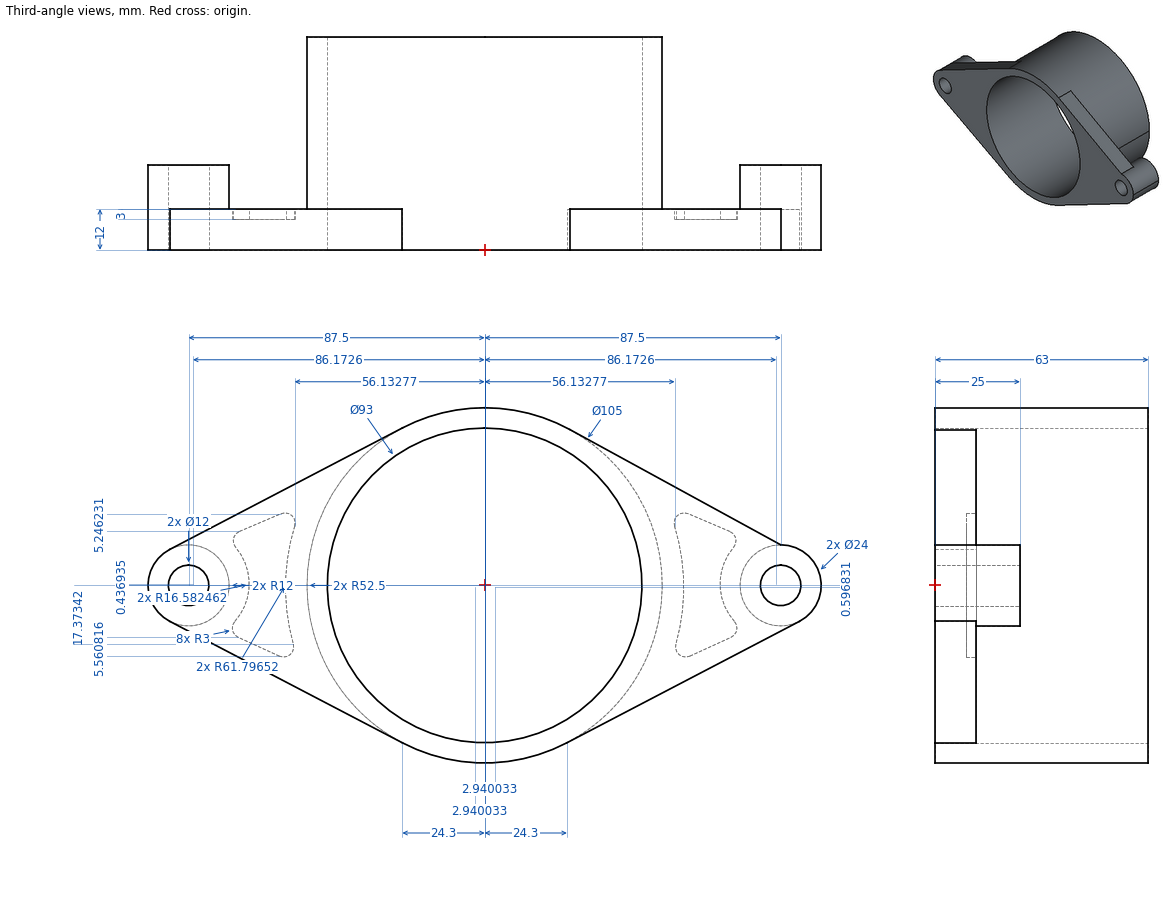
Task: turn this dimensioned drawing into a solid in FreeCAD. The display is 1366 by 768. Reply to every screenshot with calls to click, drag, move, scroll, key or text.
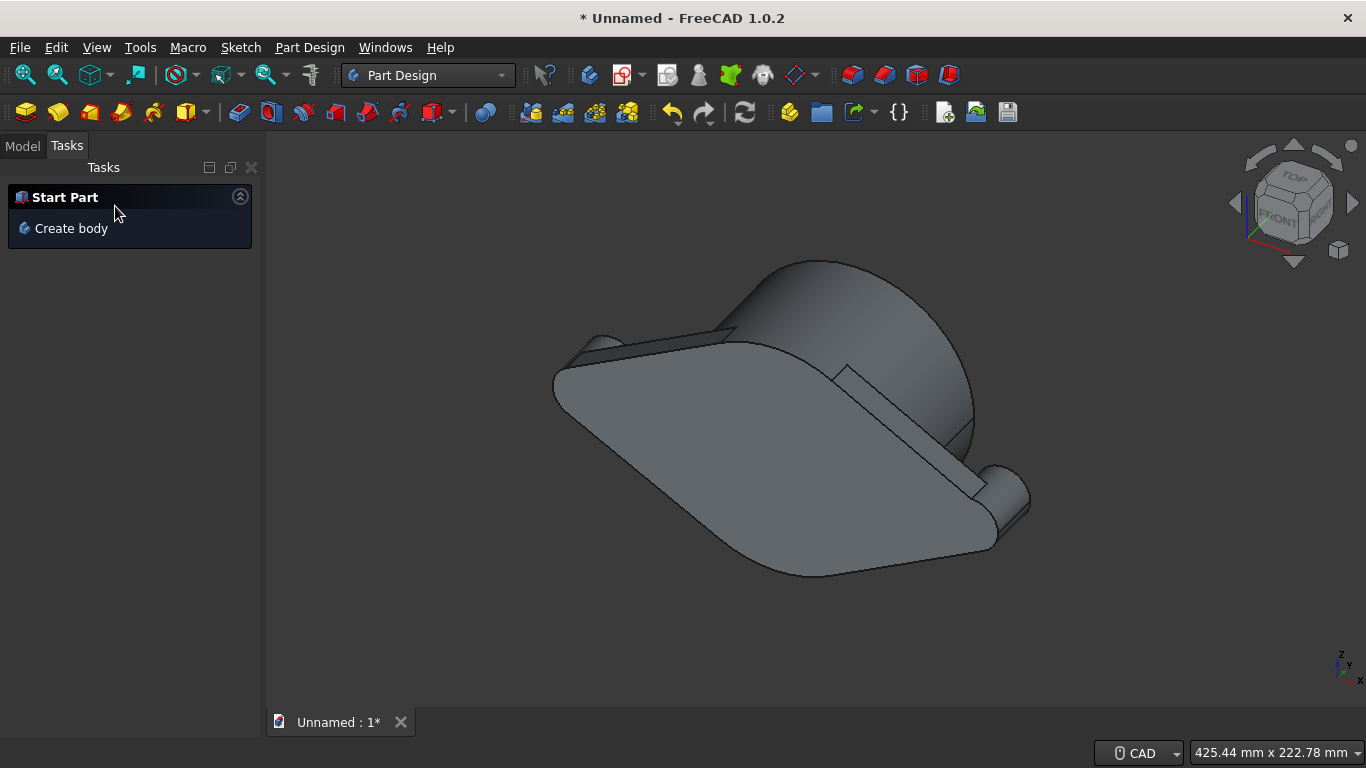
key(4)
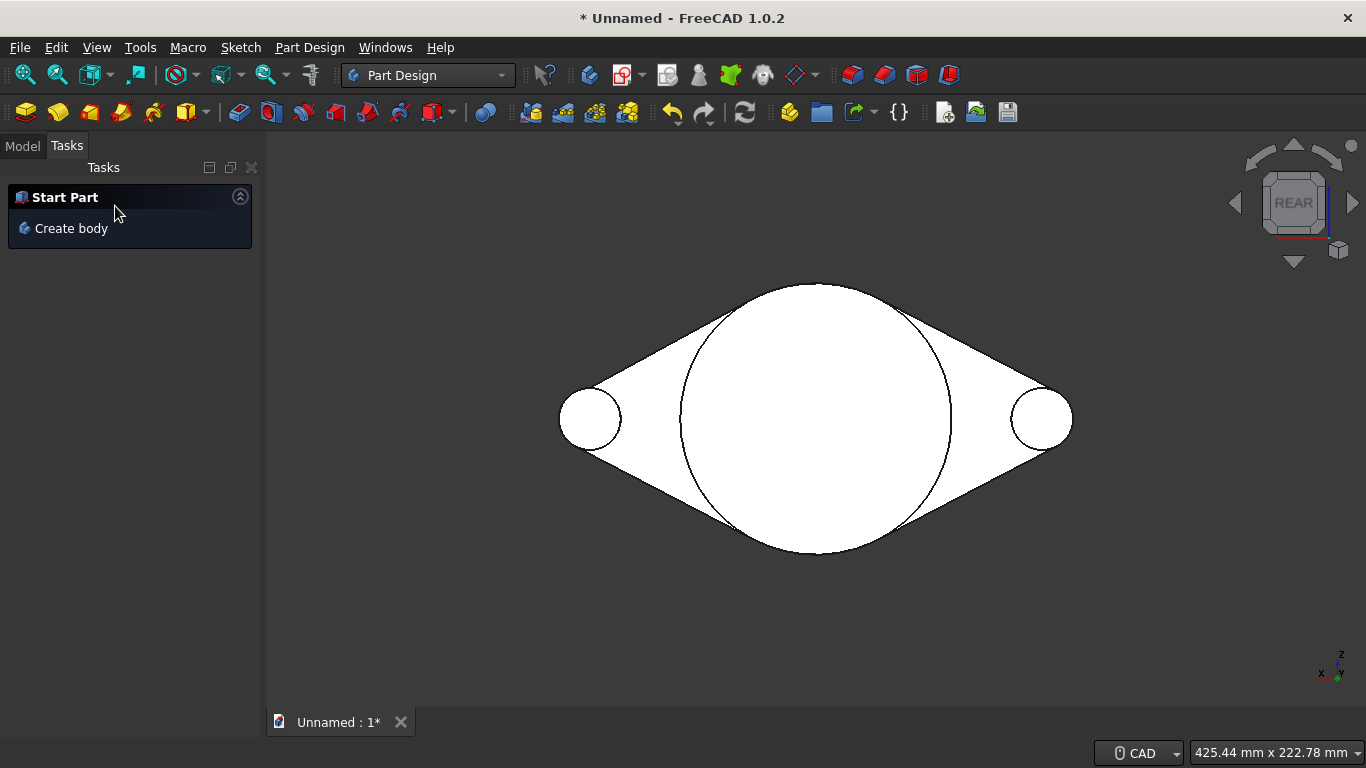
click(816, 418)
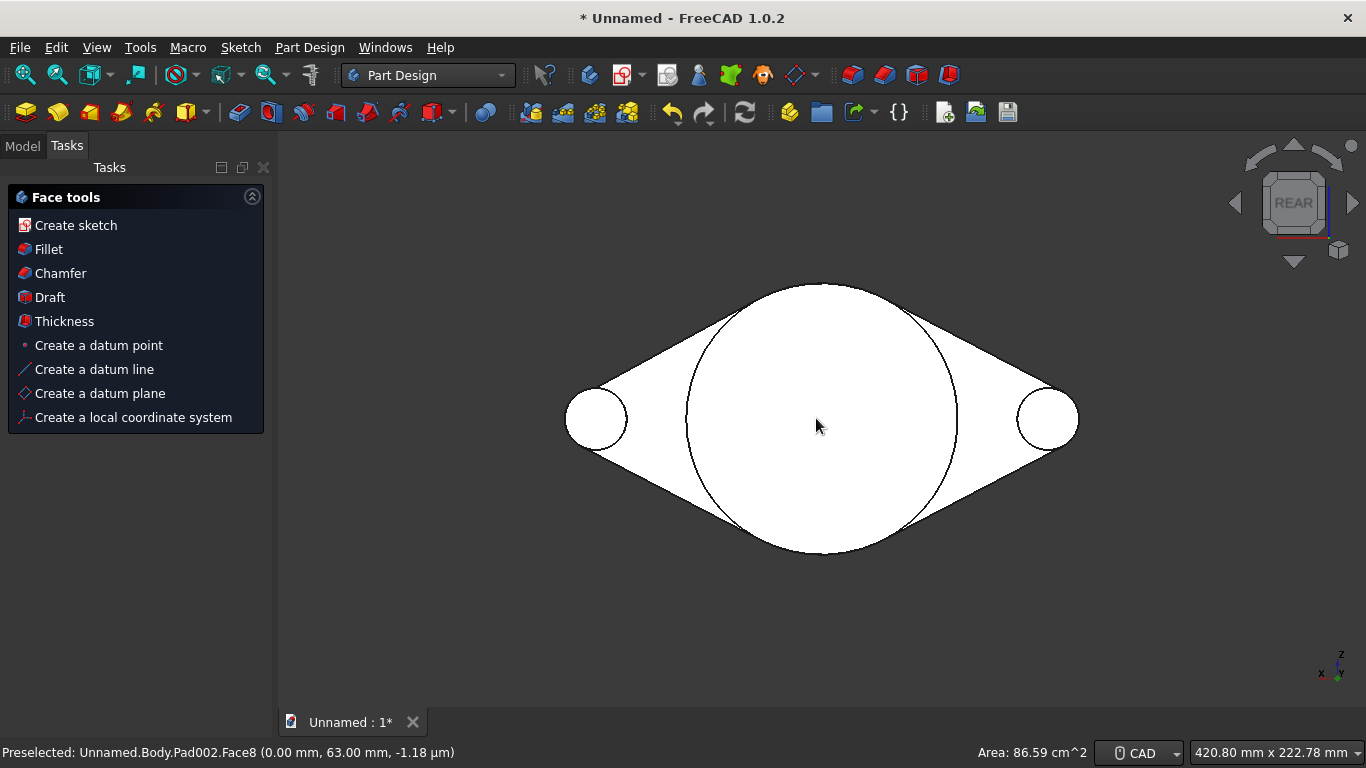
click(622, 76)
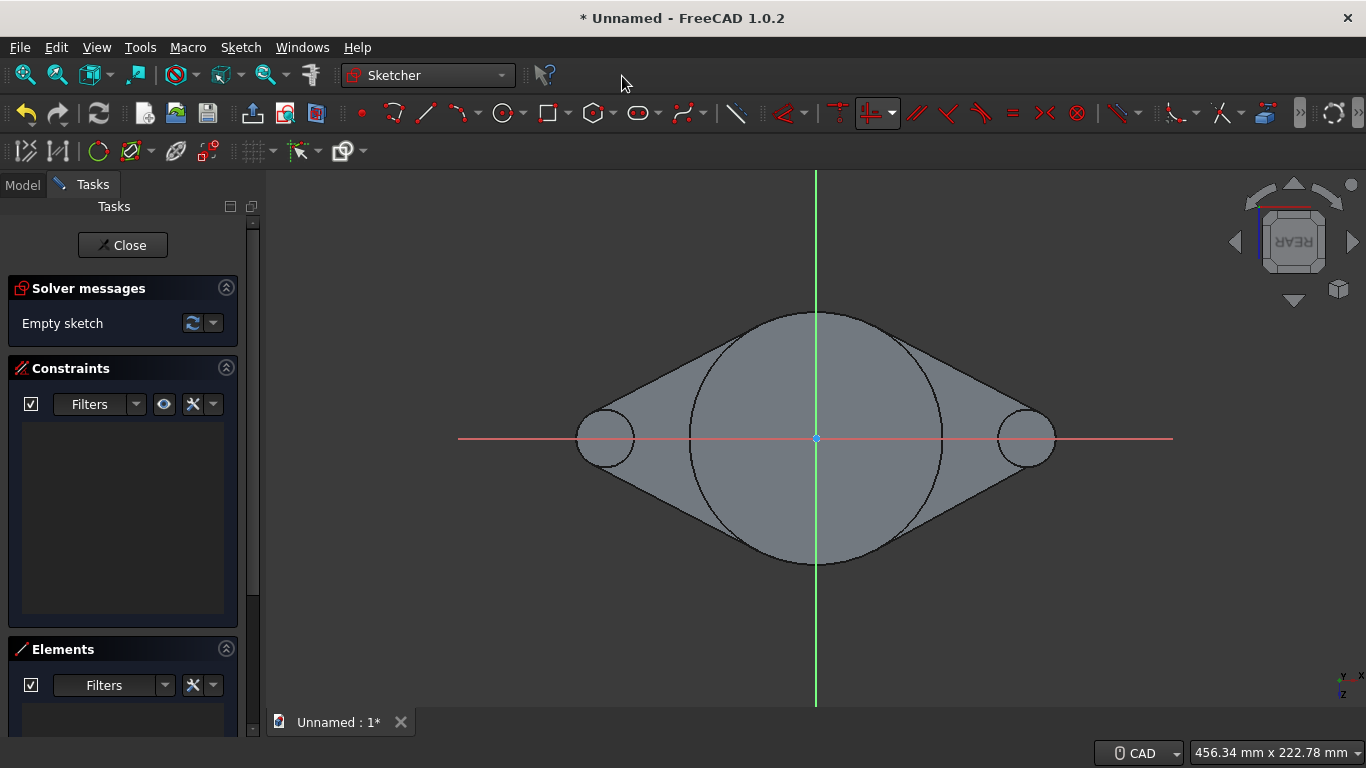
scroll(955, 439, up, 2)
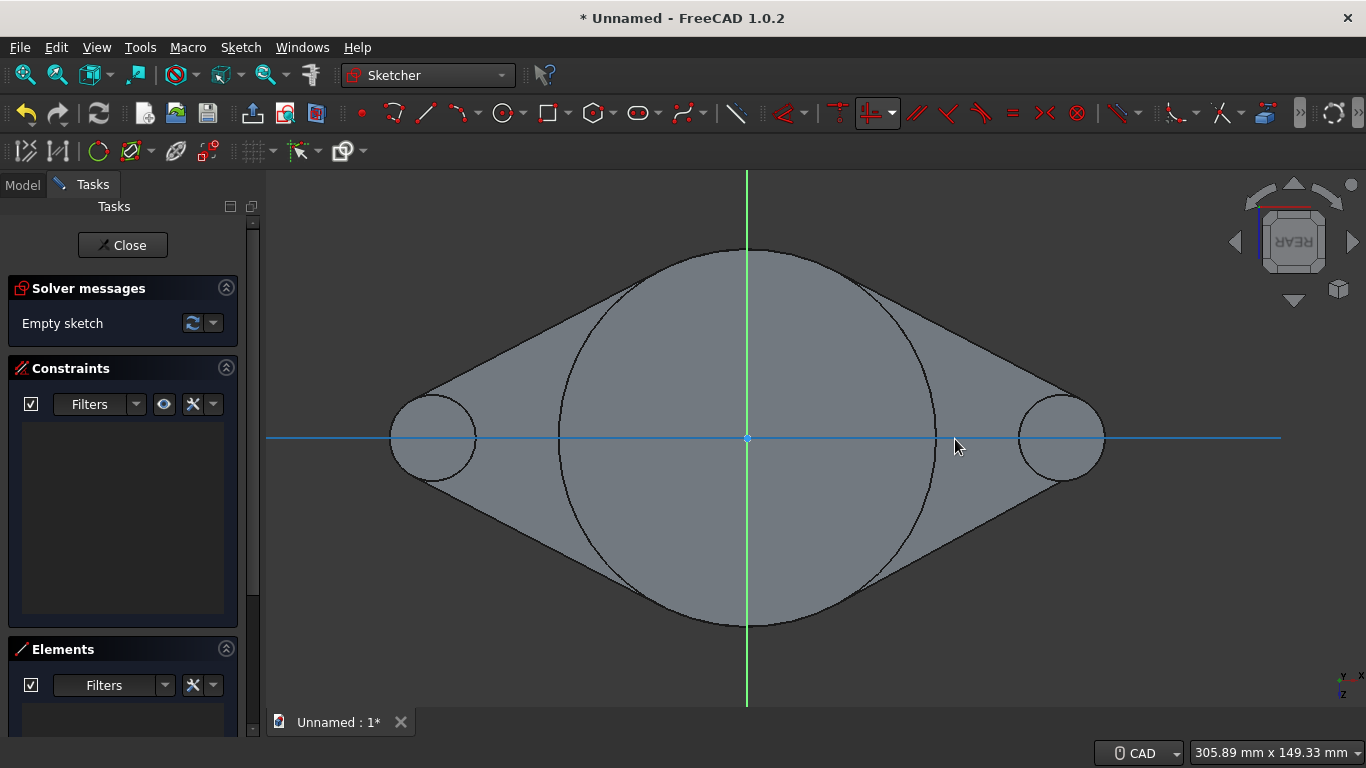
key(g)
key(c)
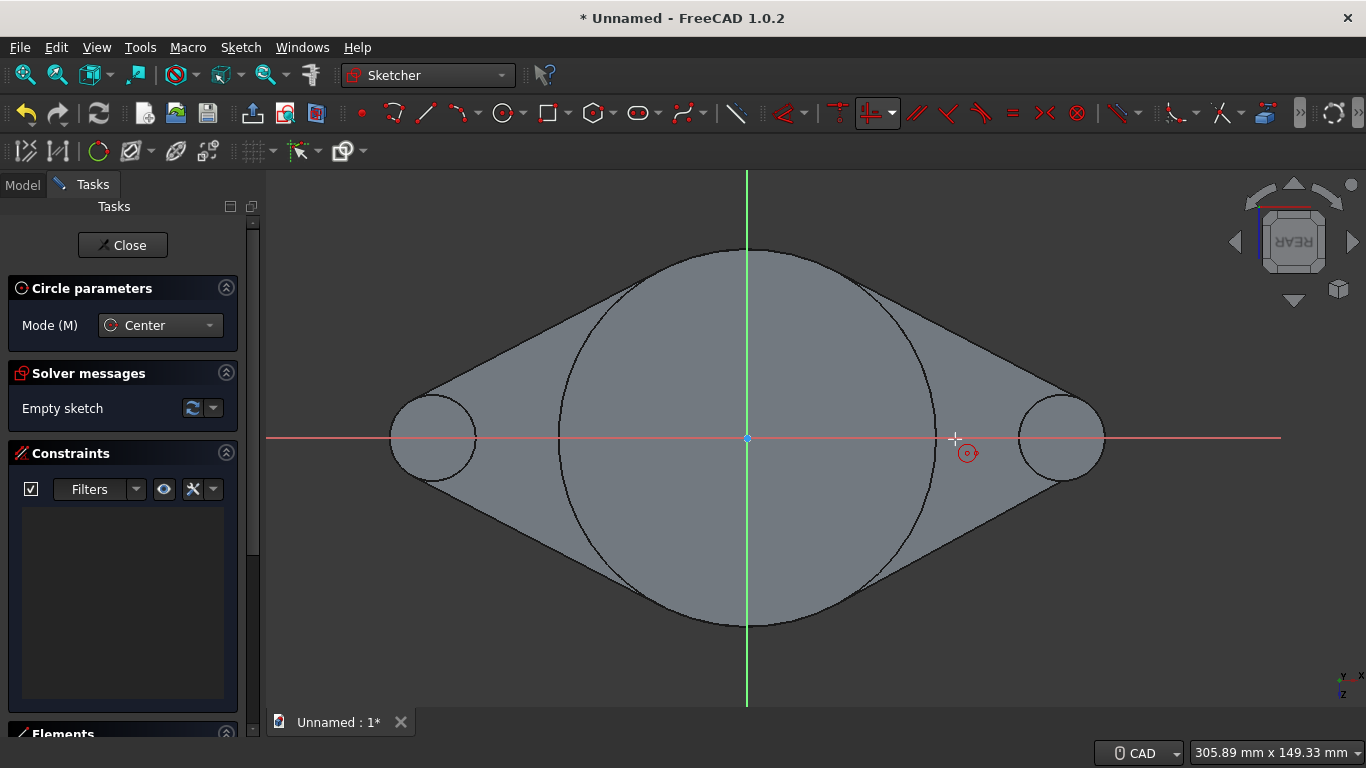
click(433, 438)
move(448, 423)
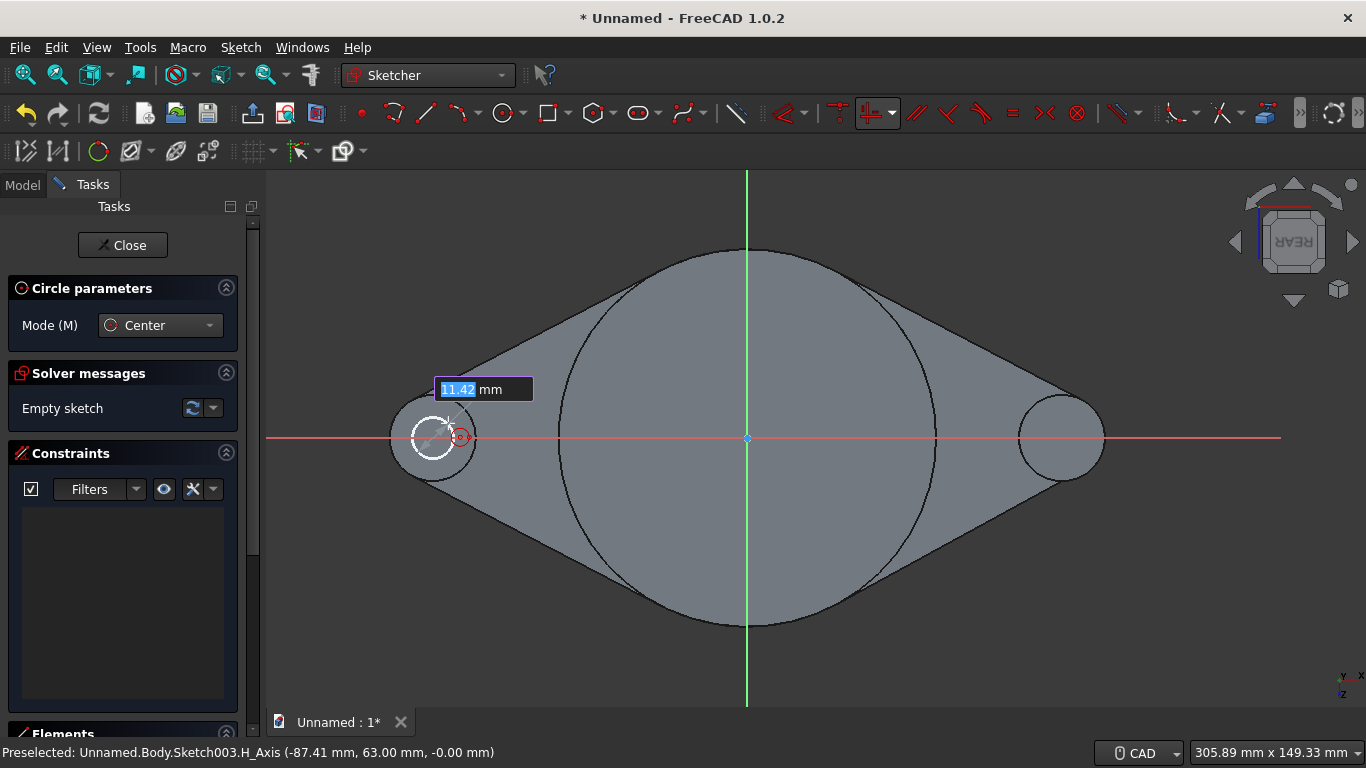
text(12)
key(Return)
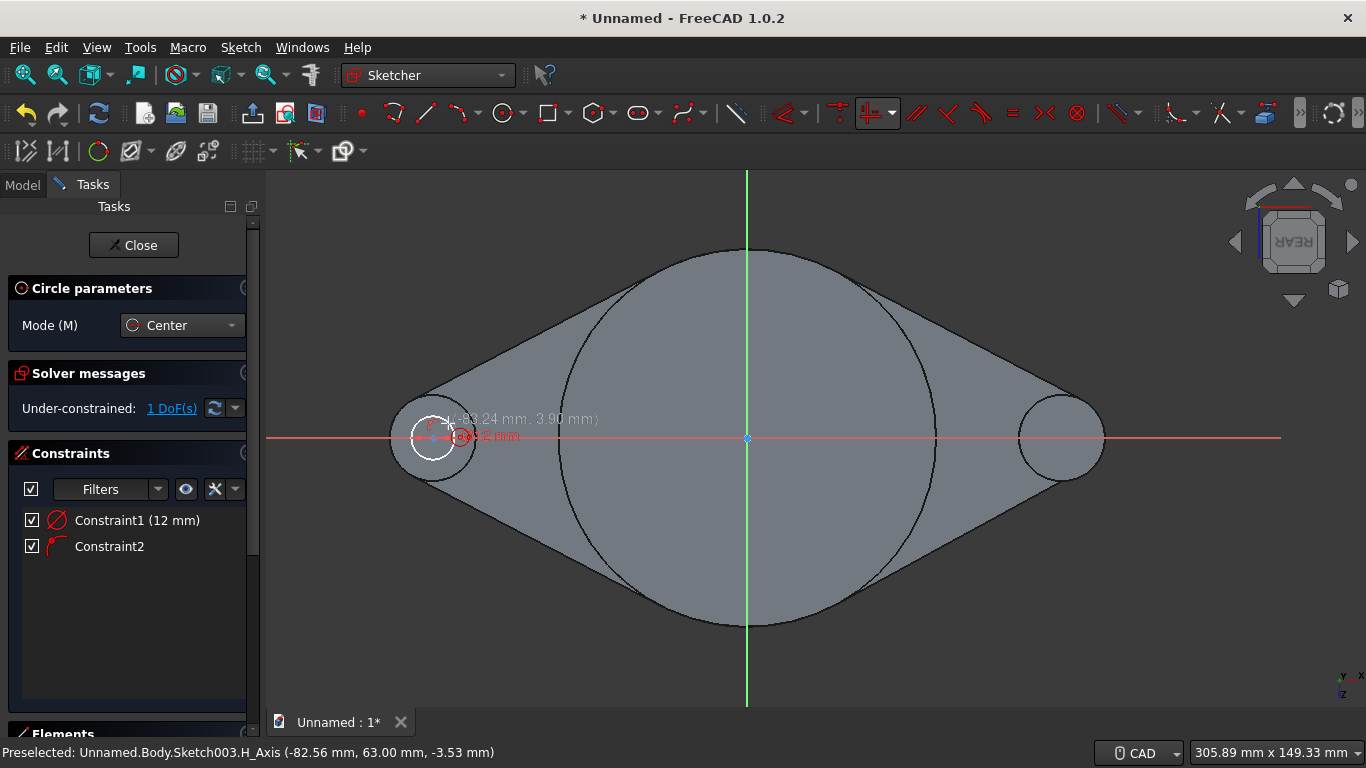
click(747, 438)
move(866, 320)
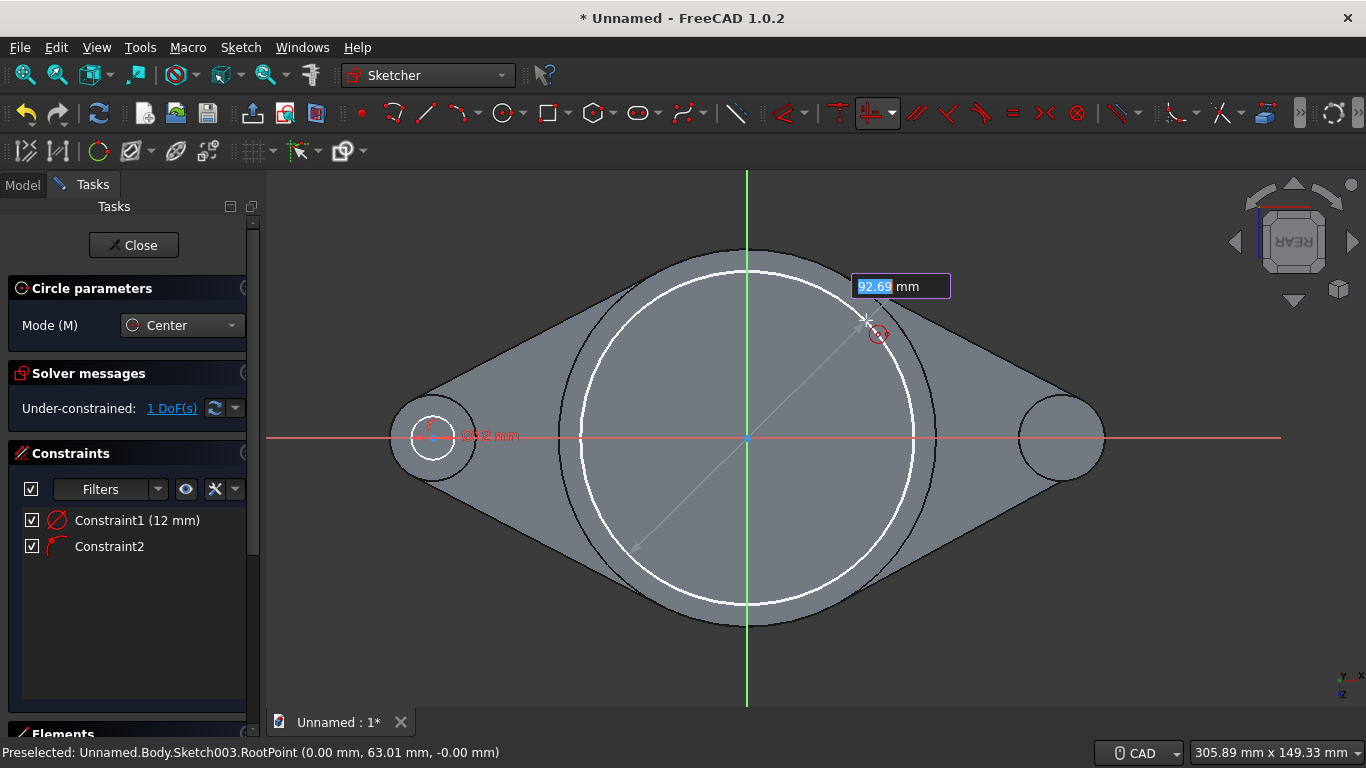
text(93)
key(Return)